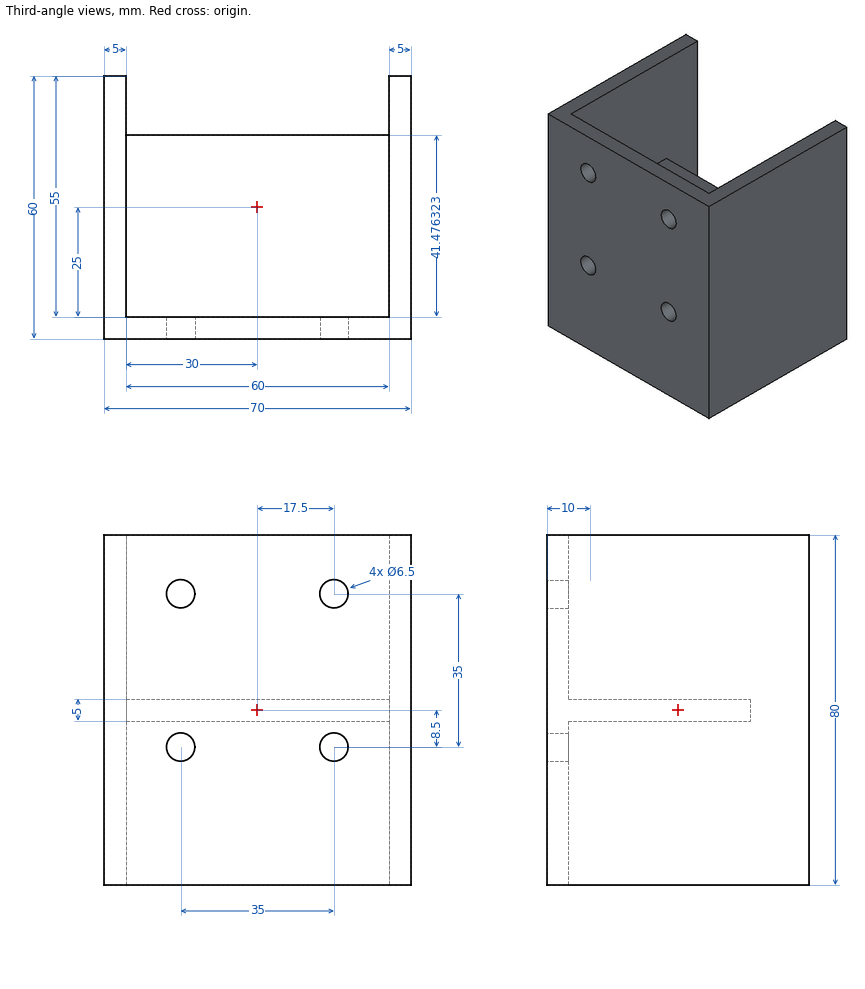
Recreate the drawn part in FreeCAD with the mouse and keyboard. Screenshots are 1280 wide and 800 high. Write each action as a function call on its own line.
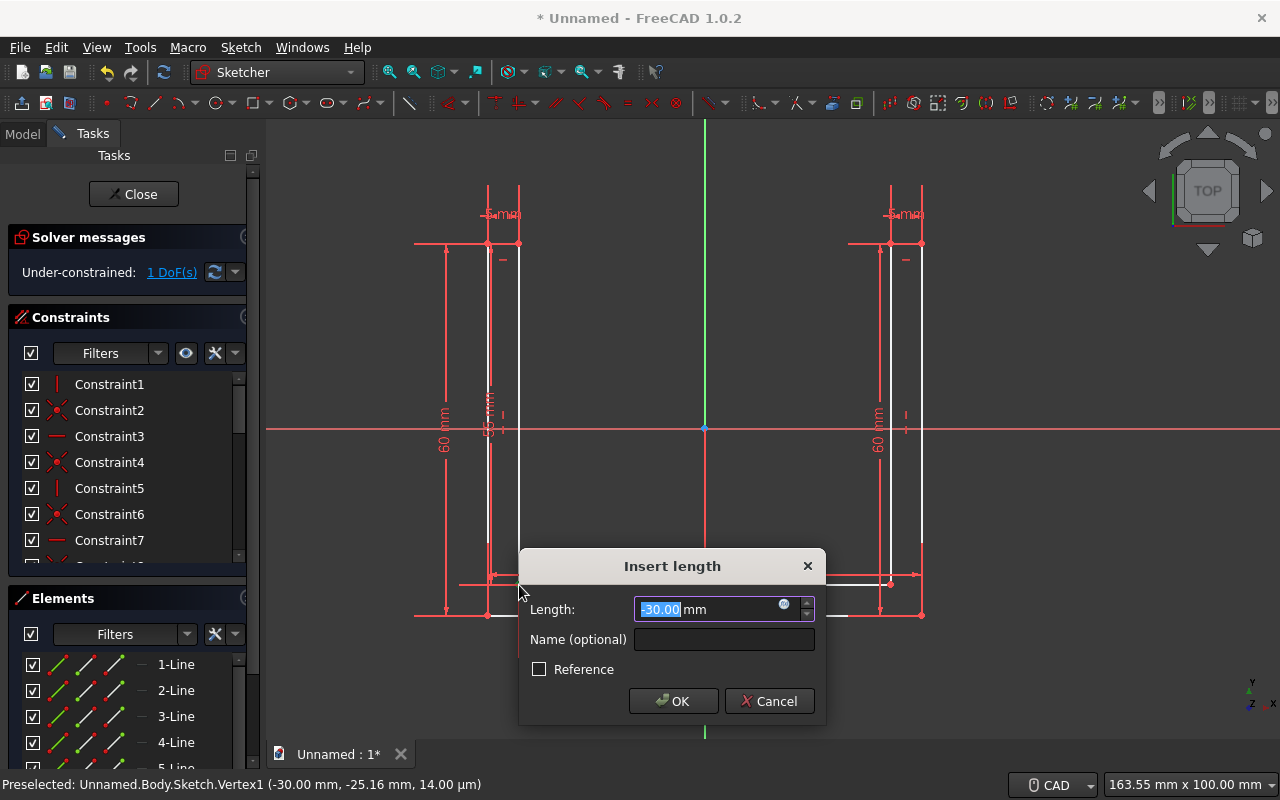
text(-30)
key(Return)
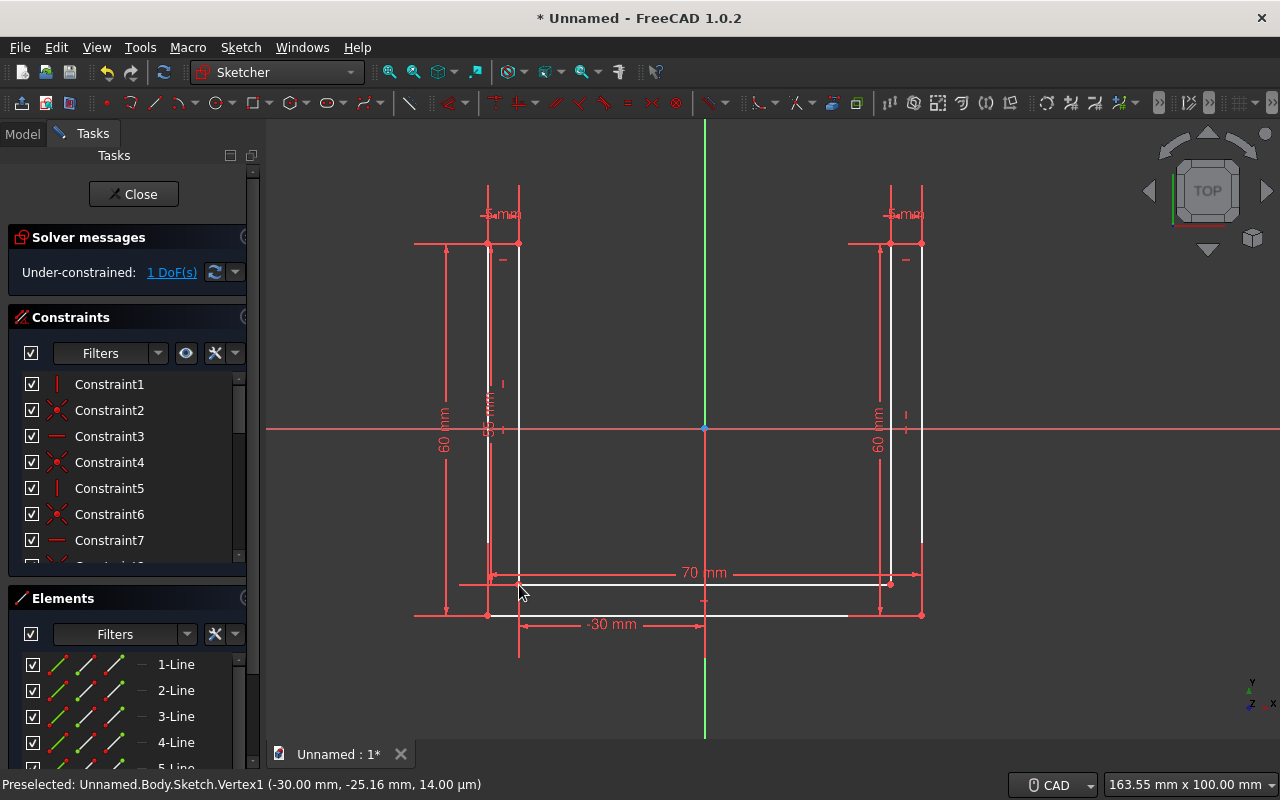
click(519, 585)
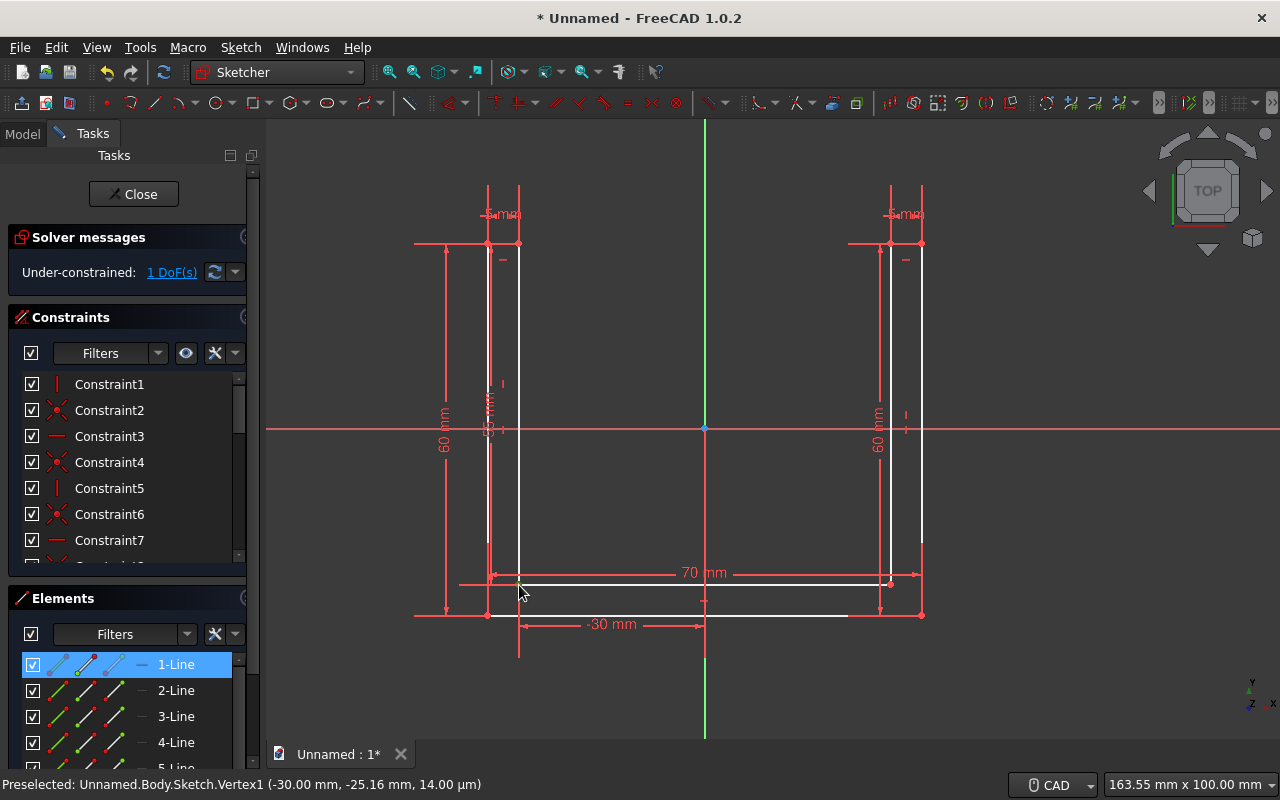
key(i)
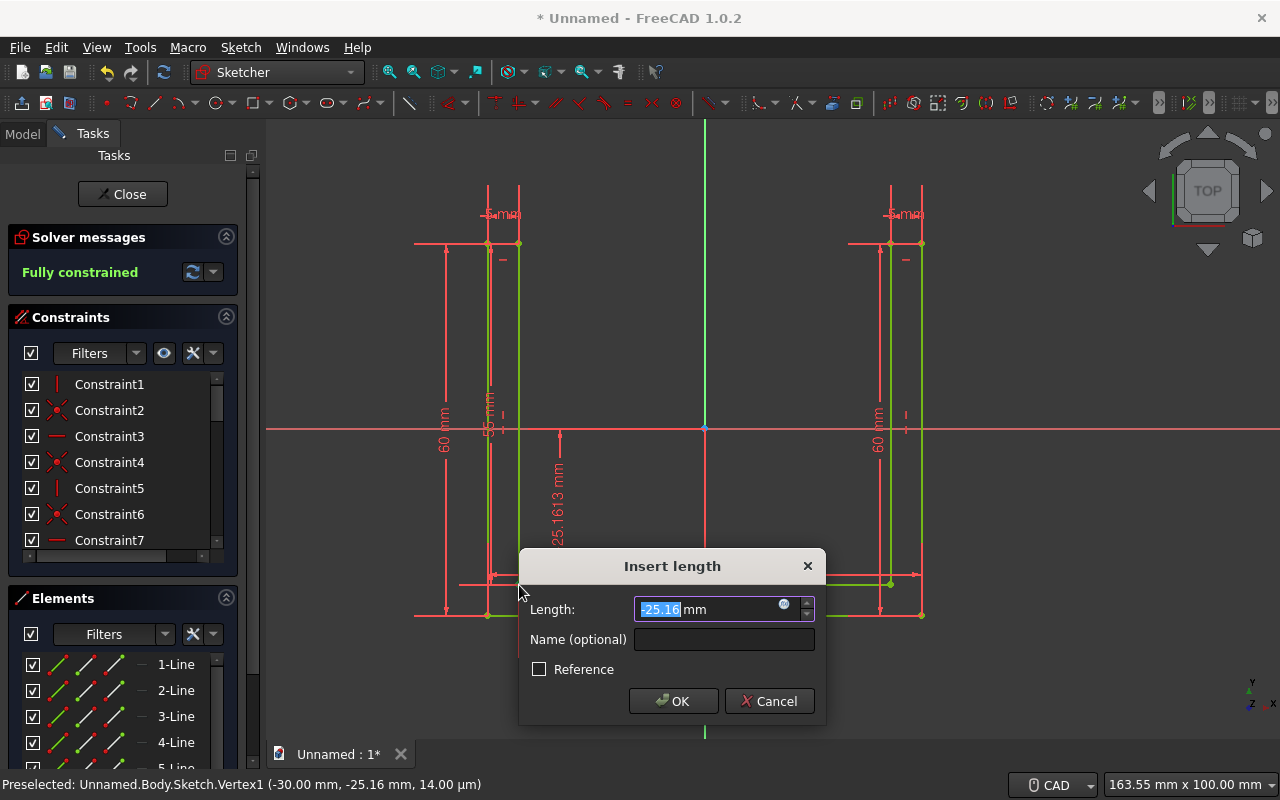
text(-25)
key(Return)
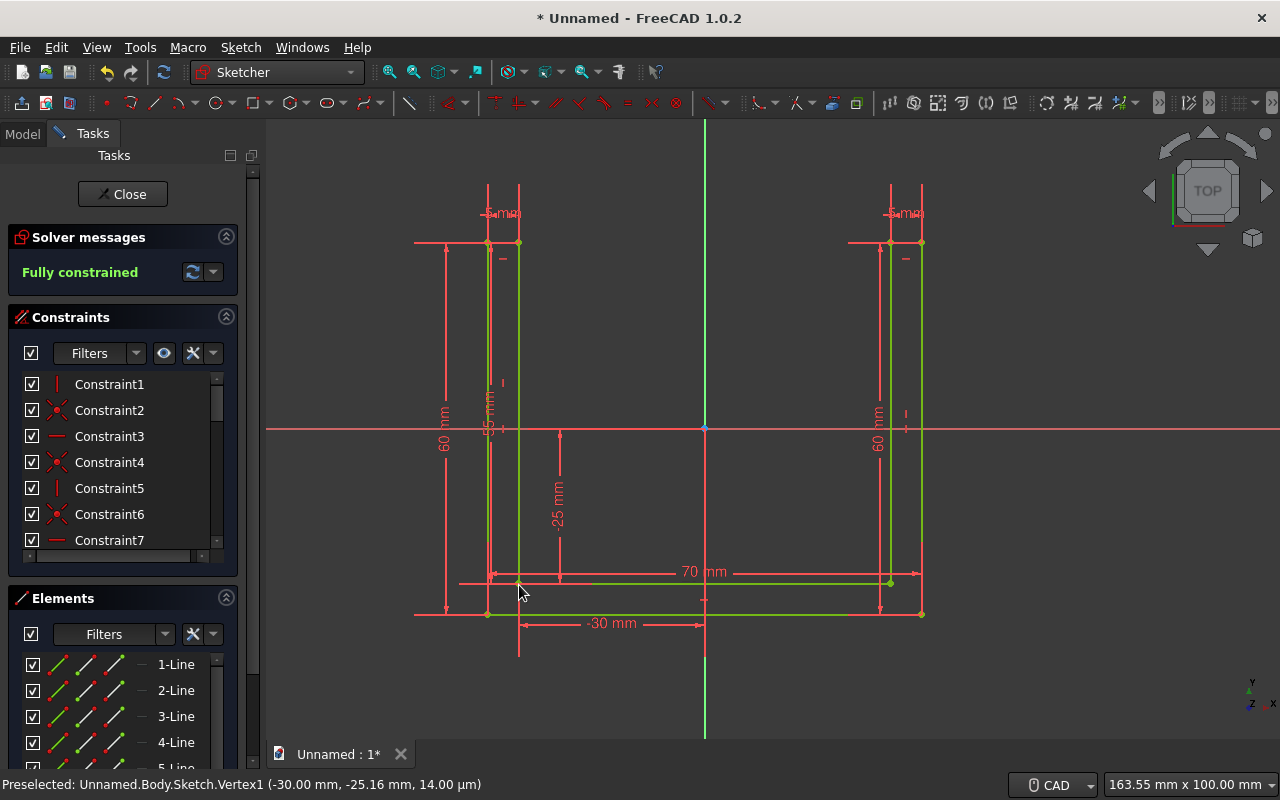
click(123, 194)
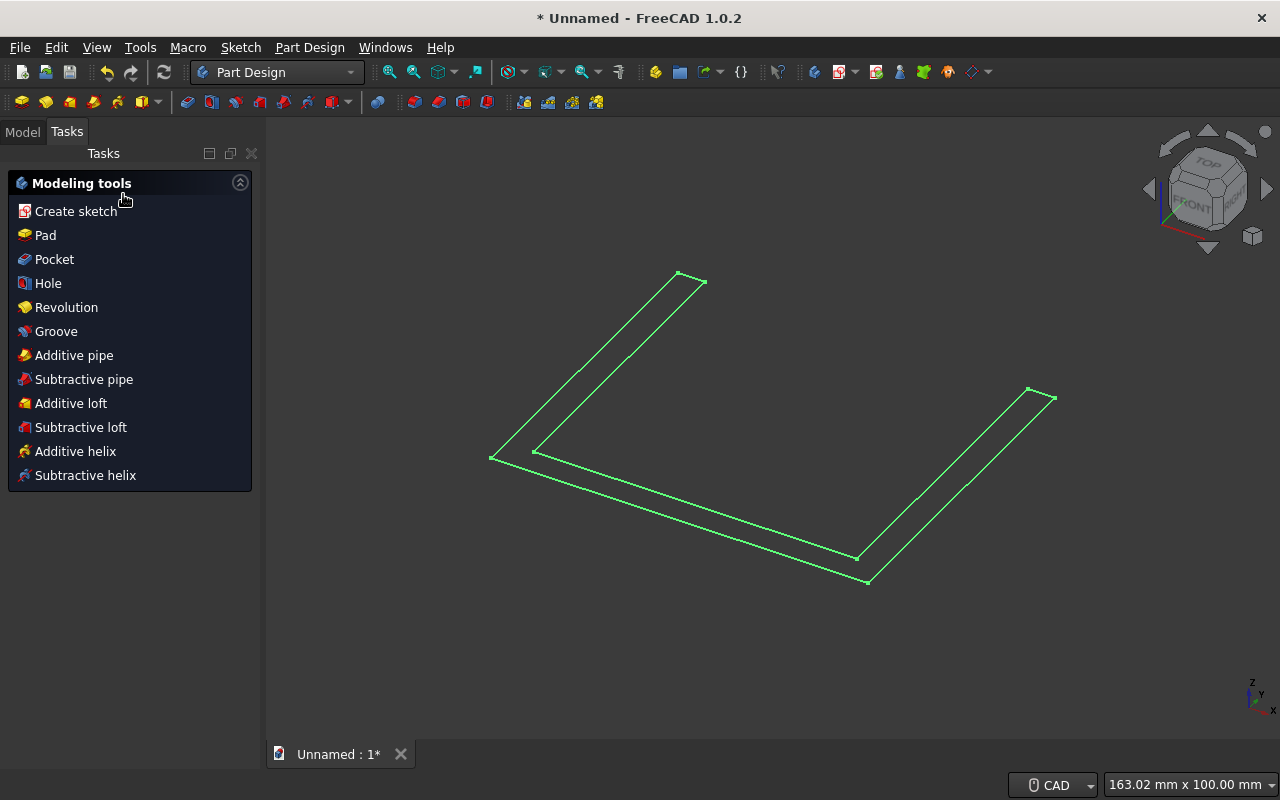
click(22, 102)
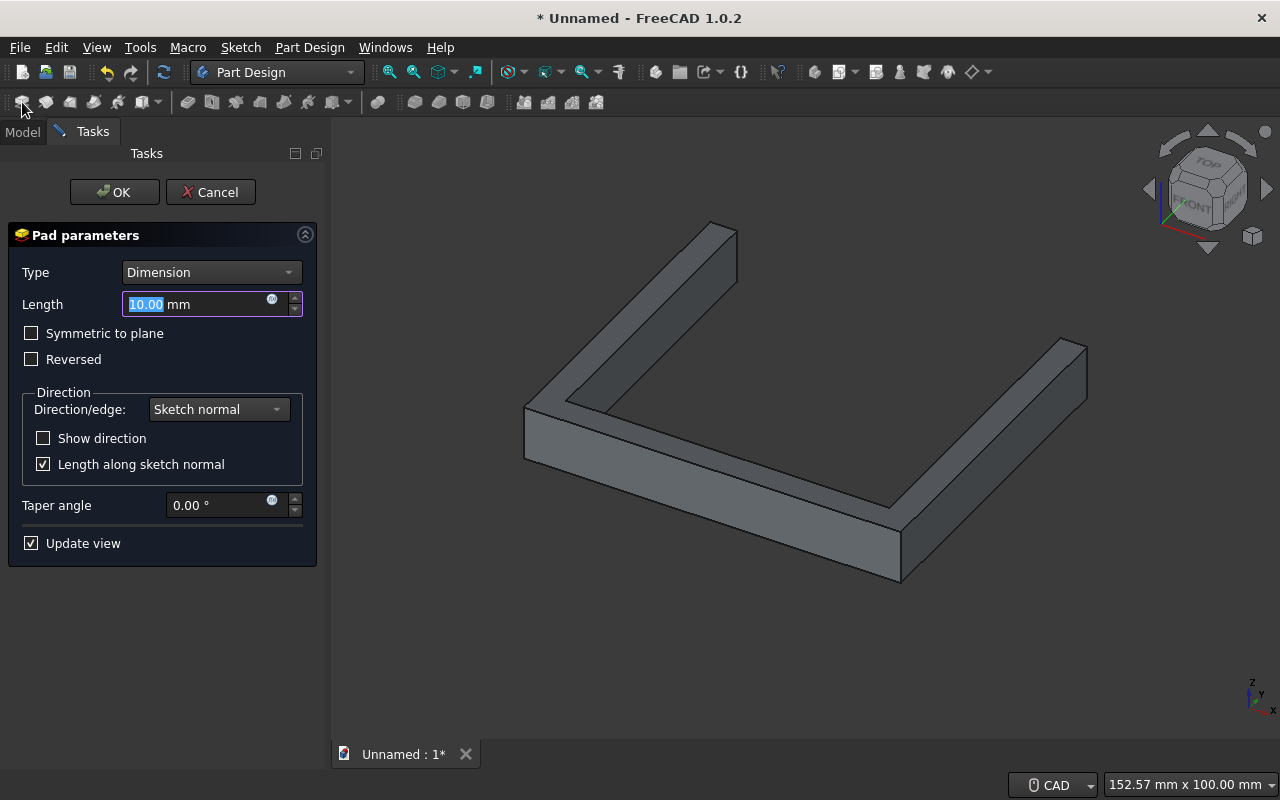
text(80)
key(Tab)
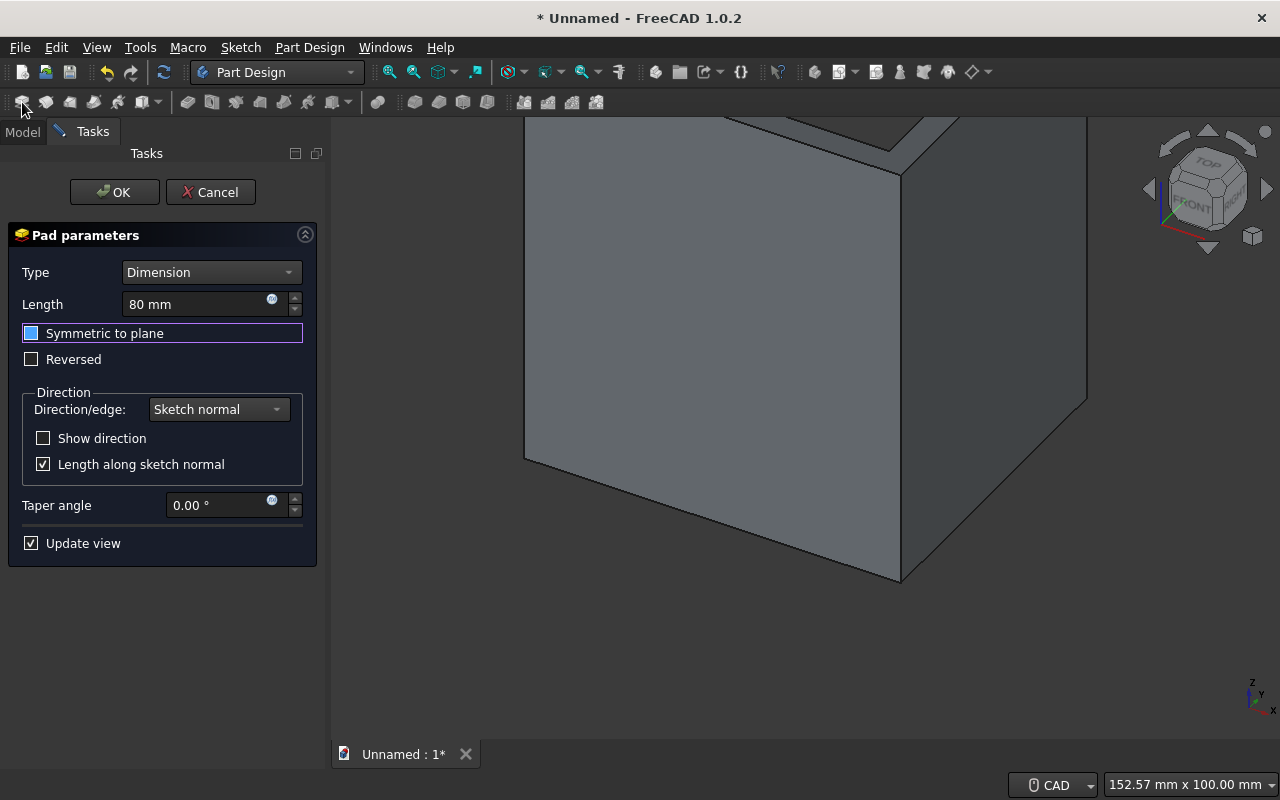
click(30, 333)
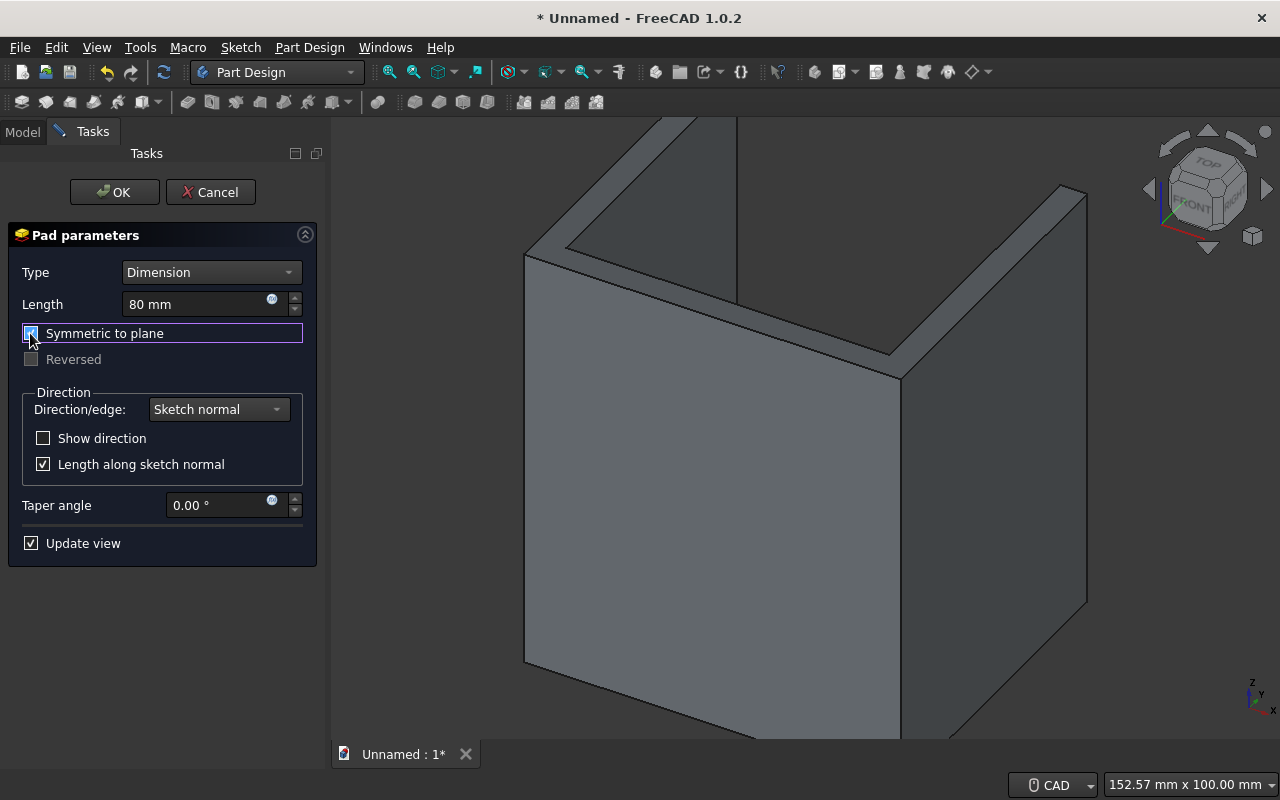
click(115, 192)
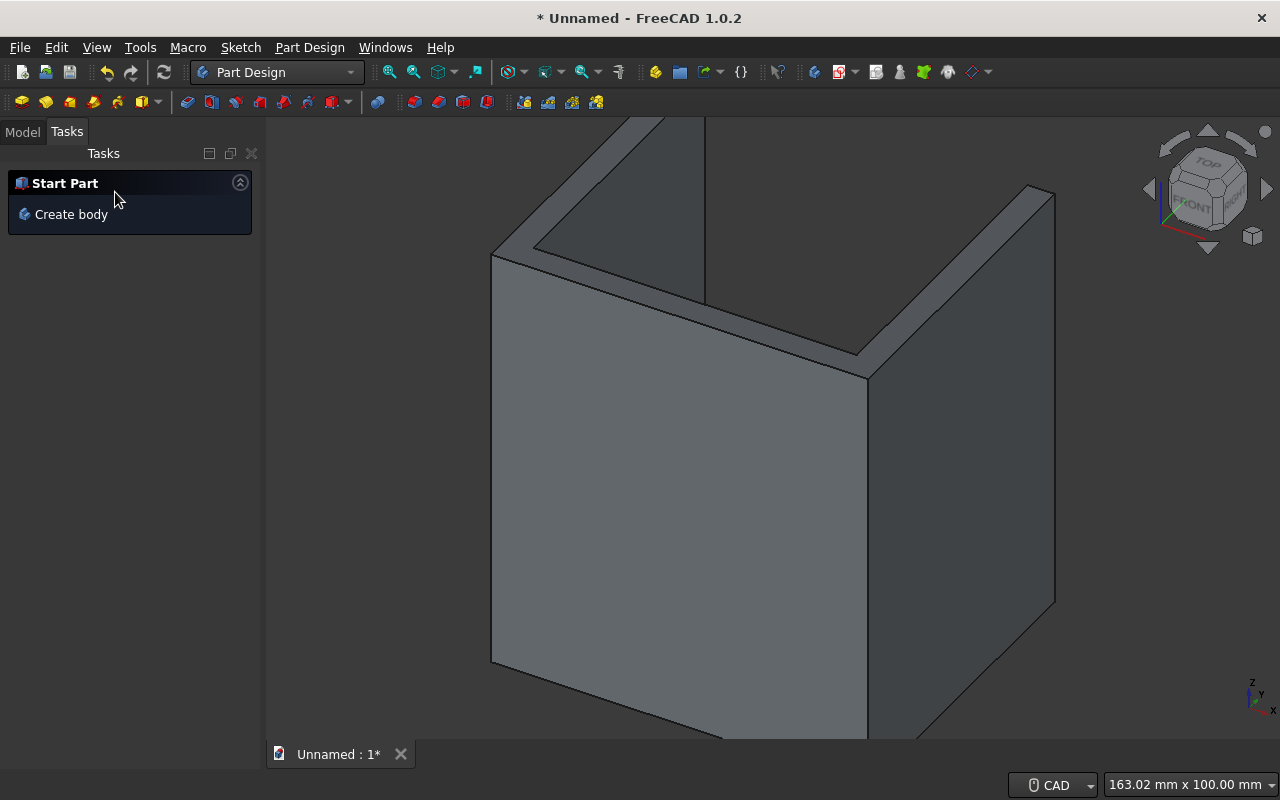
click(390, 72)